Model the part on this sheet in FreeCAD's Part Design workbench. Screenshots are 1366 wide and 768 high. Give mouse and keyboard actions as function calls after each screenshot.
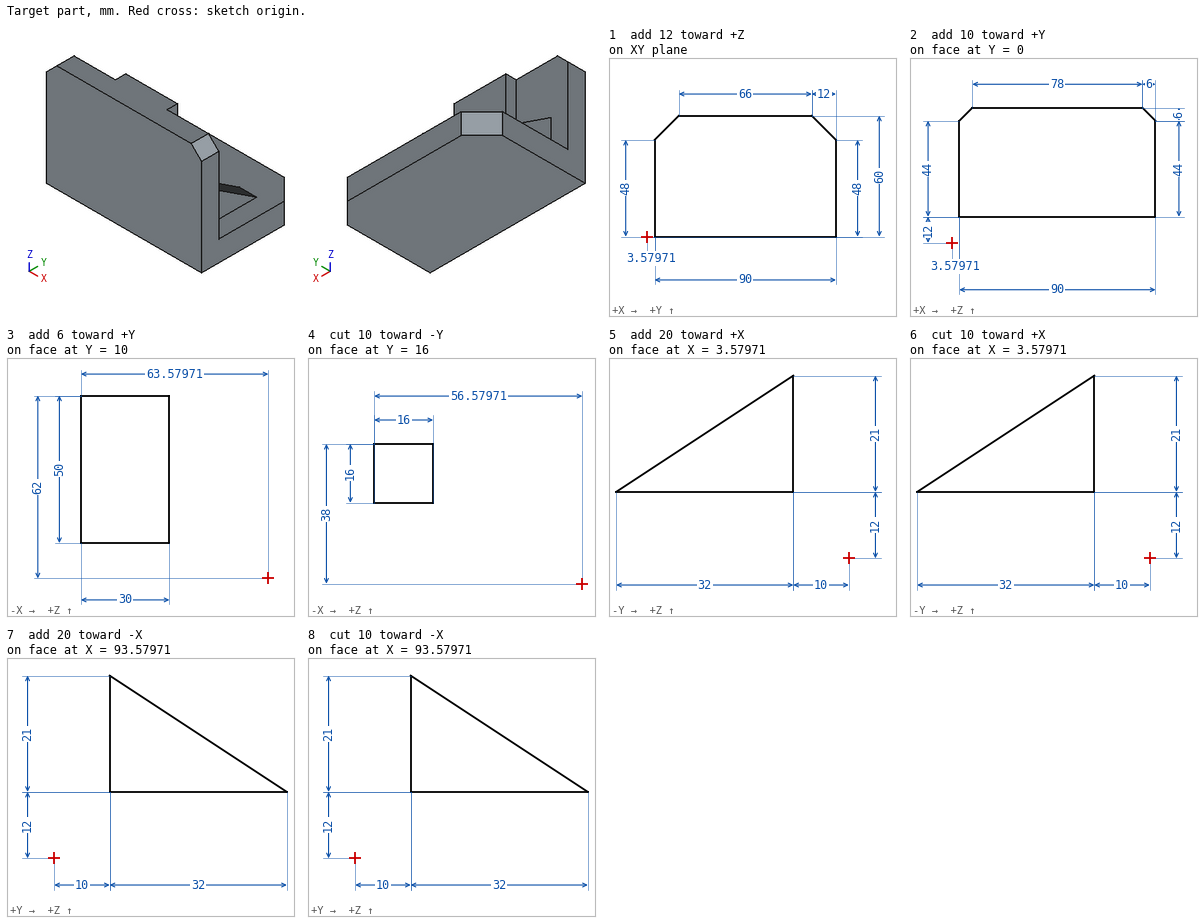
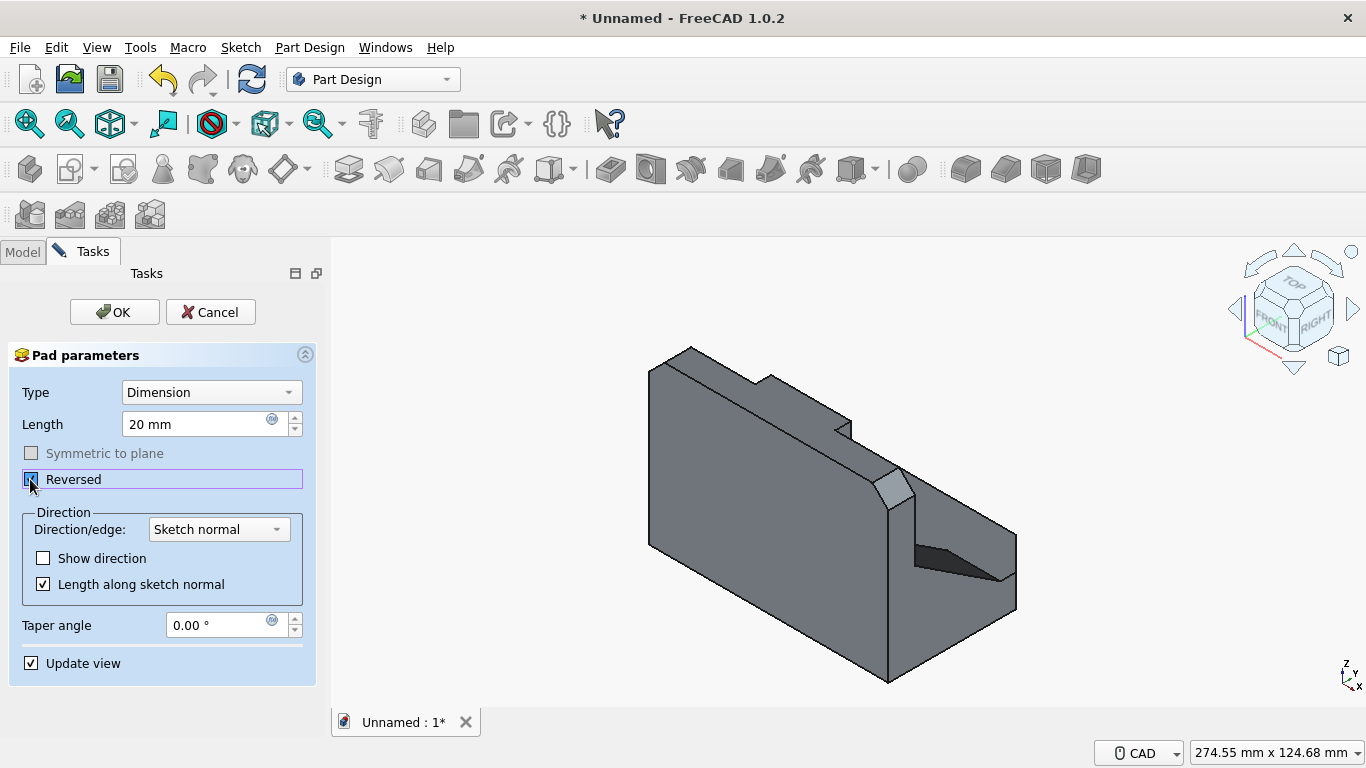
click(115, 312)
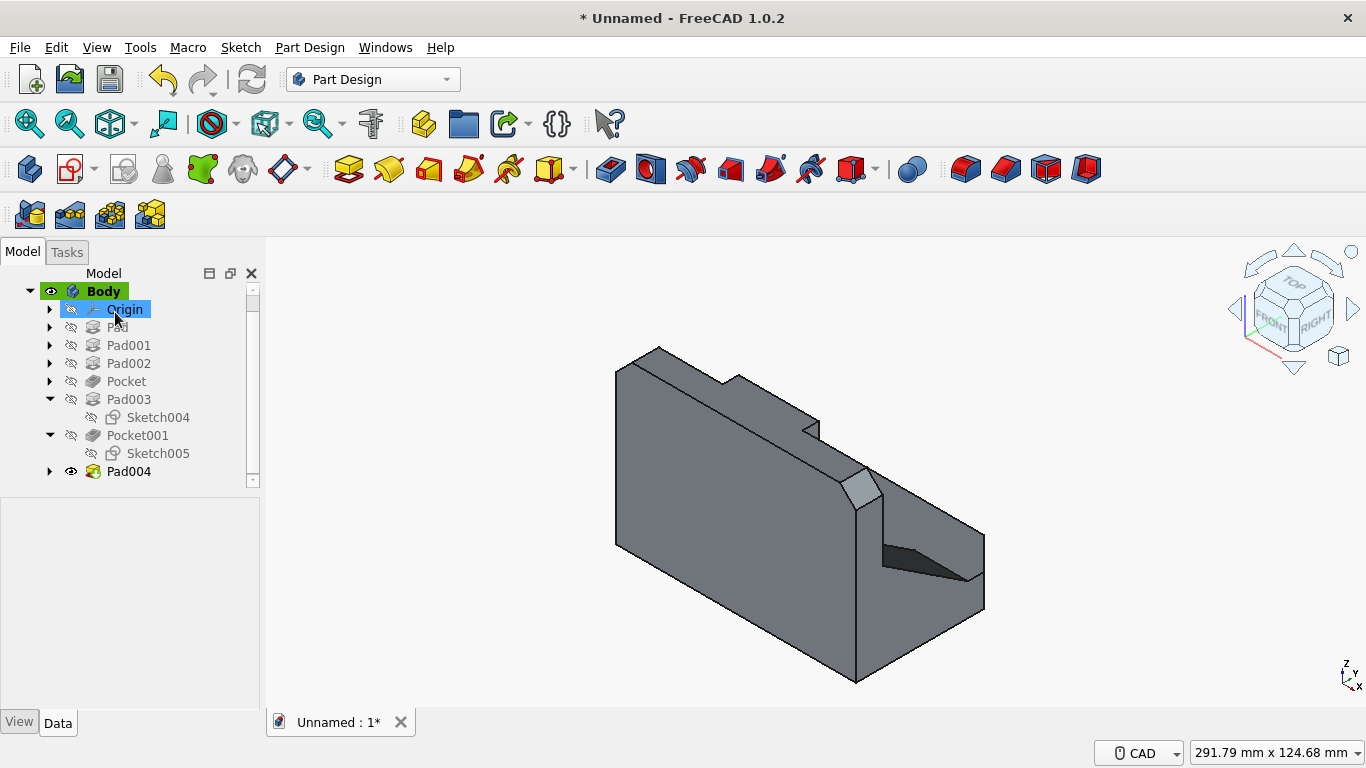
click(902, 619)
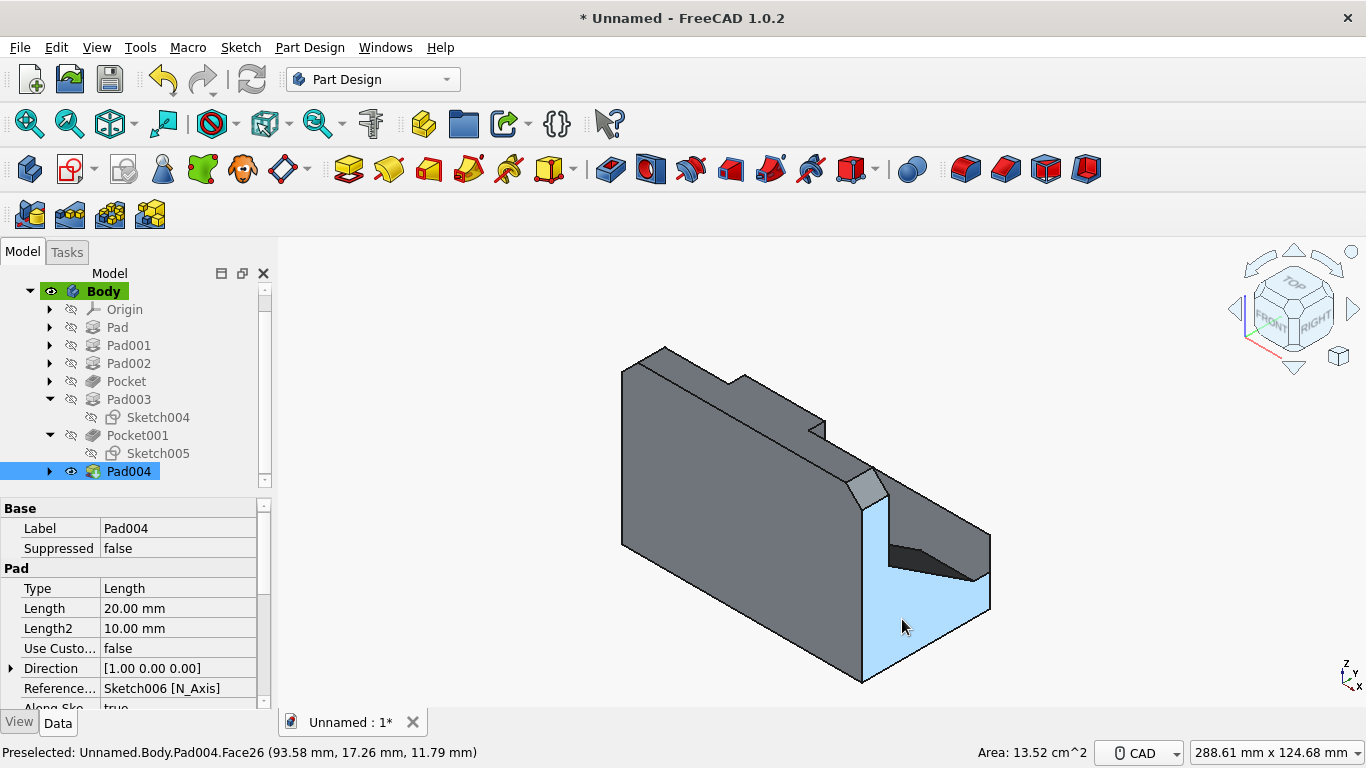
click(70, 170)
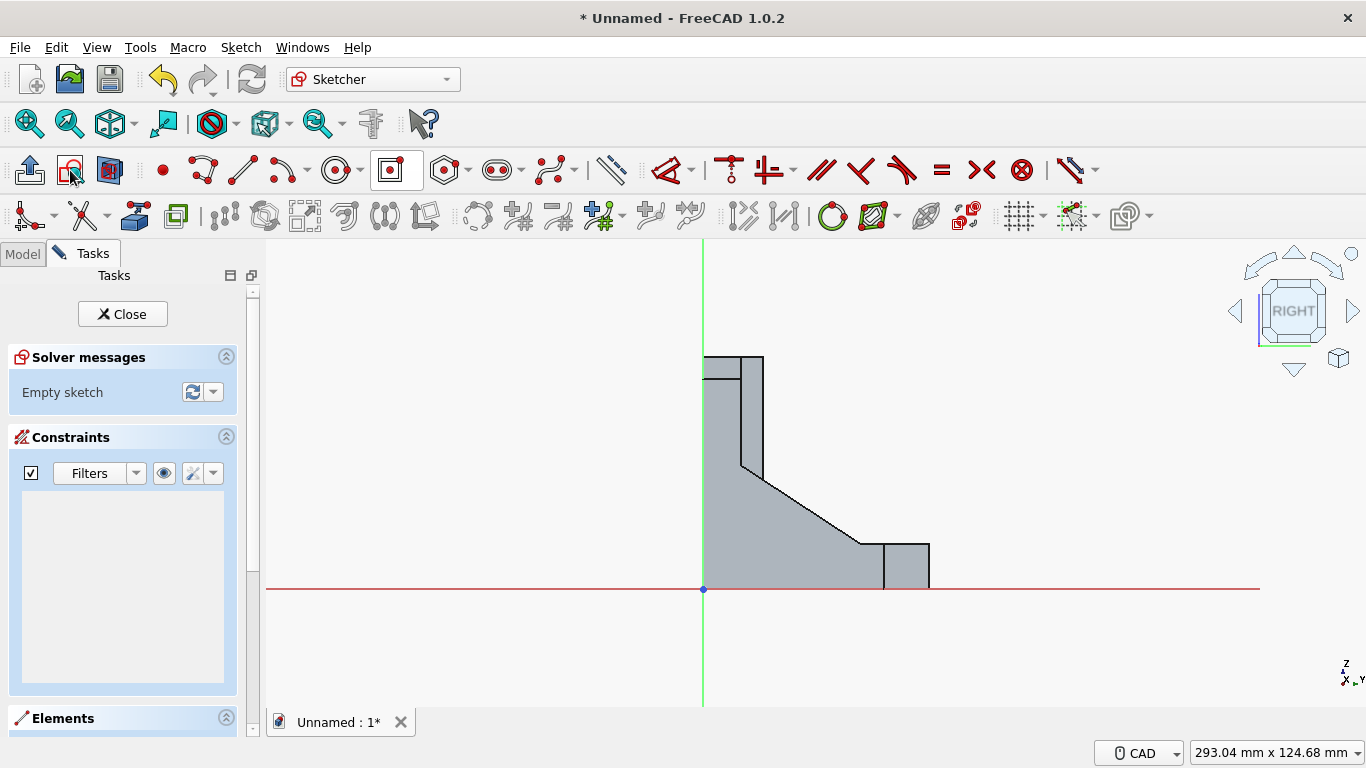
scroll(811, 572, up, 4)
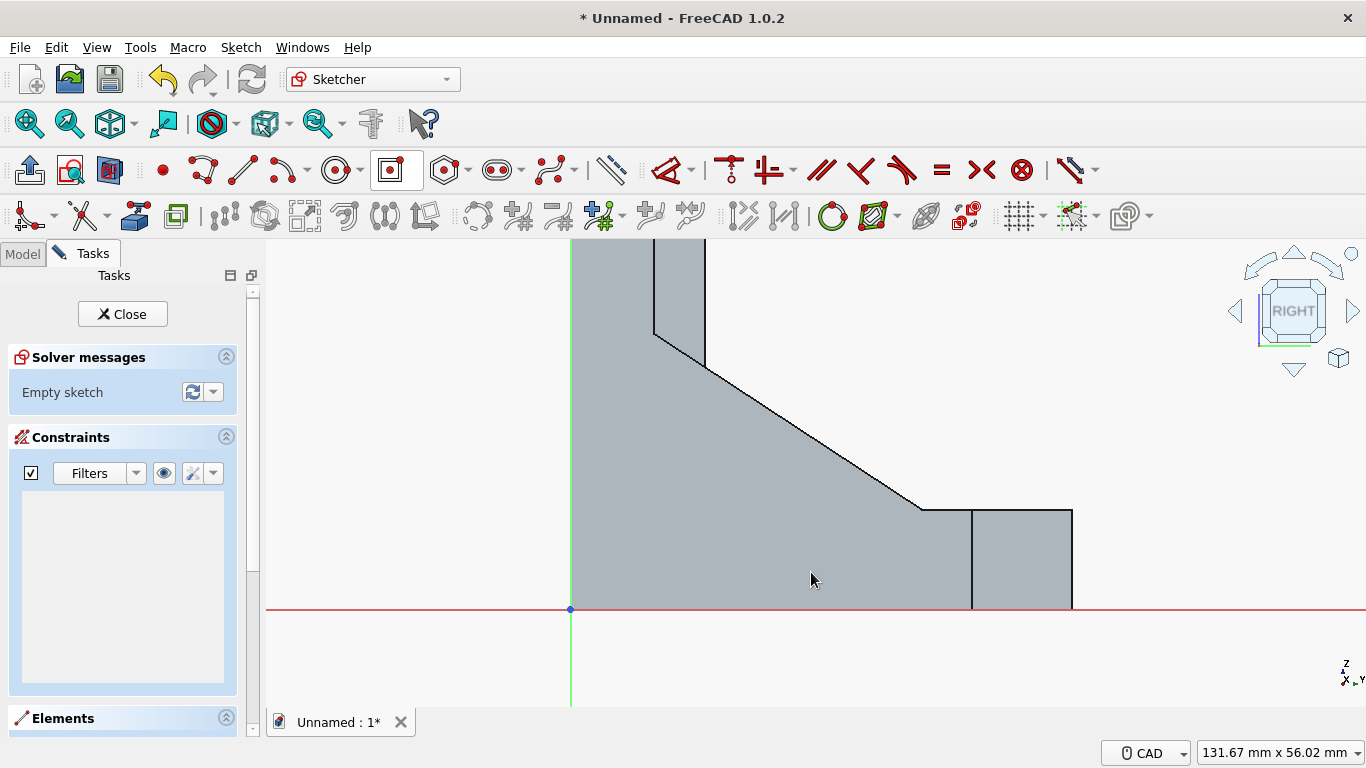
click(204, 170)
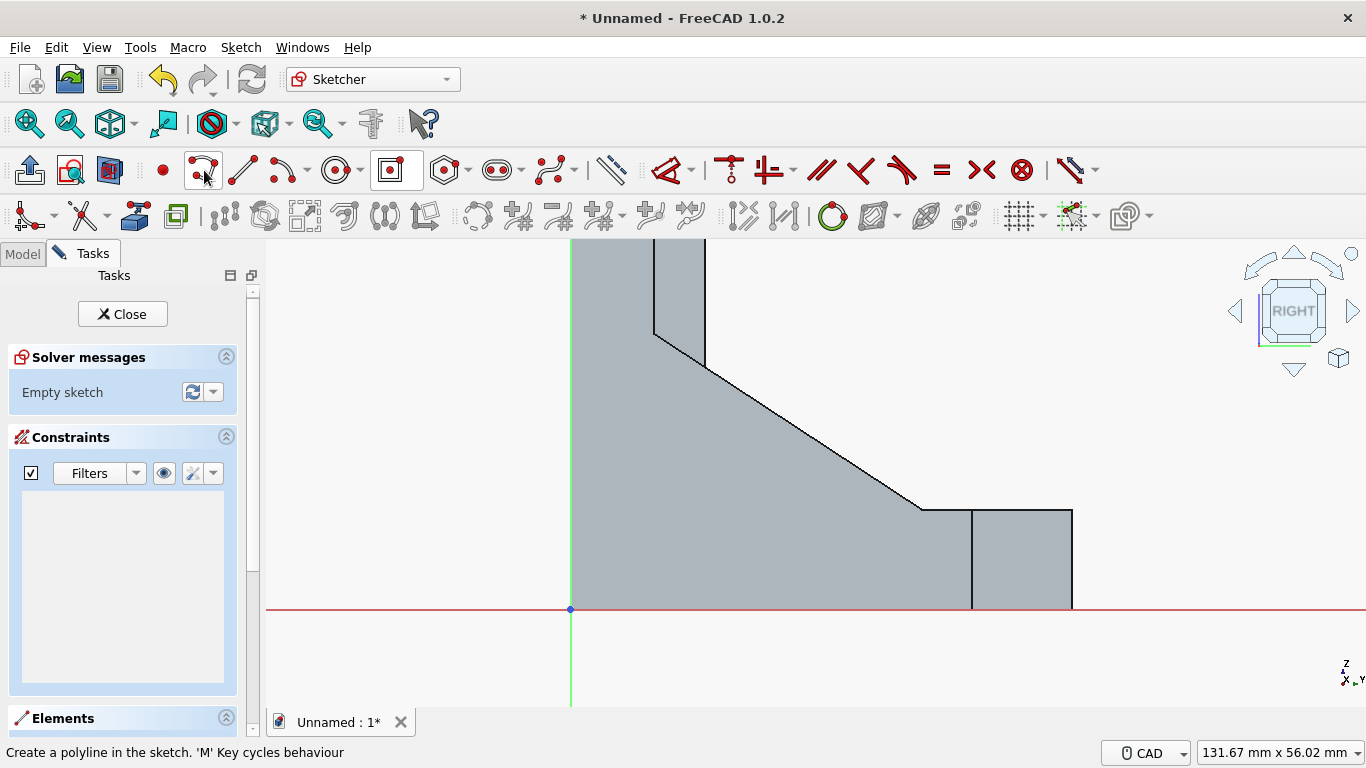
click(654, 510)
click(922, 510)
click(654, 334)
click(654, 511)
key(Escape)
key(Escape)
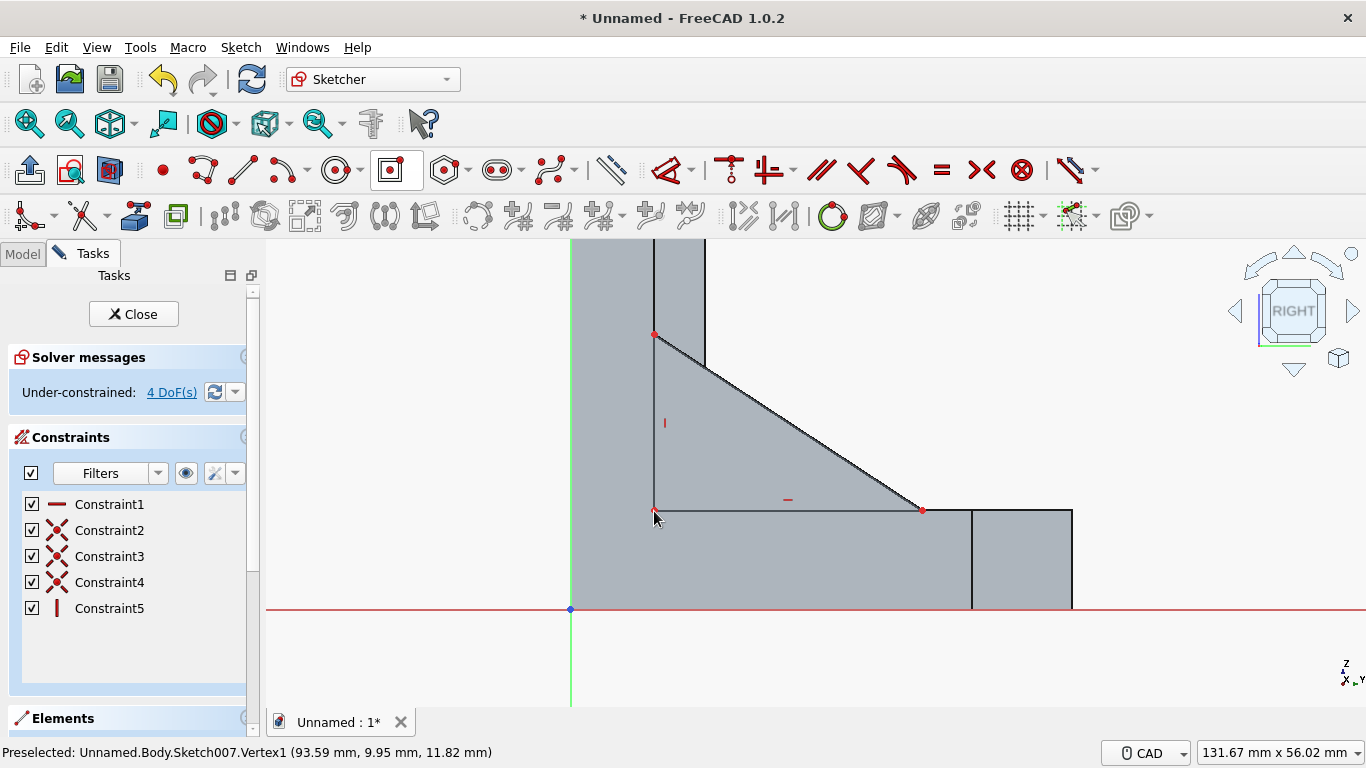
click(666, 170)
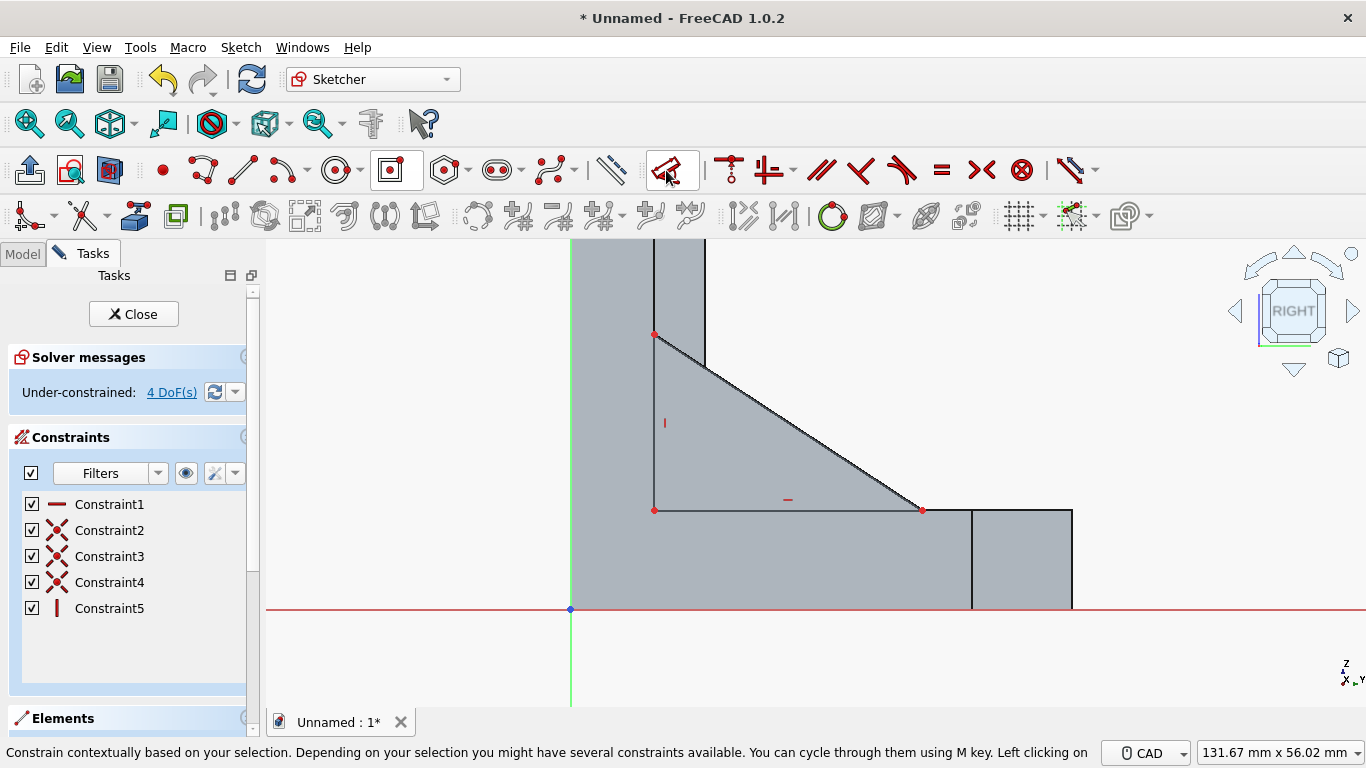
click(734, 511)
click(788, 545)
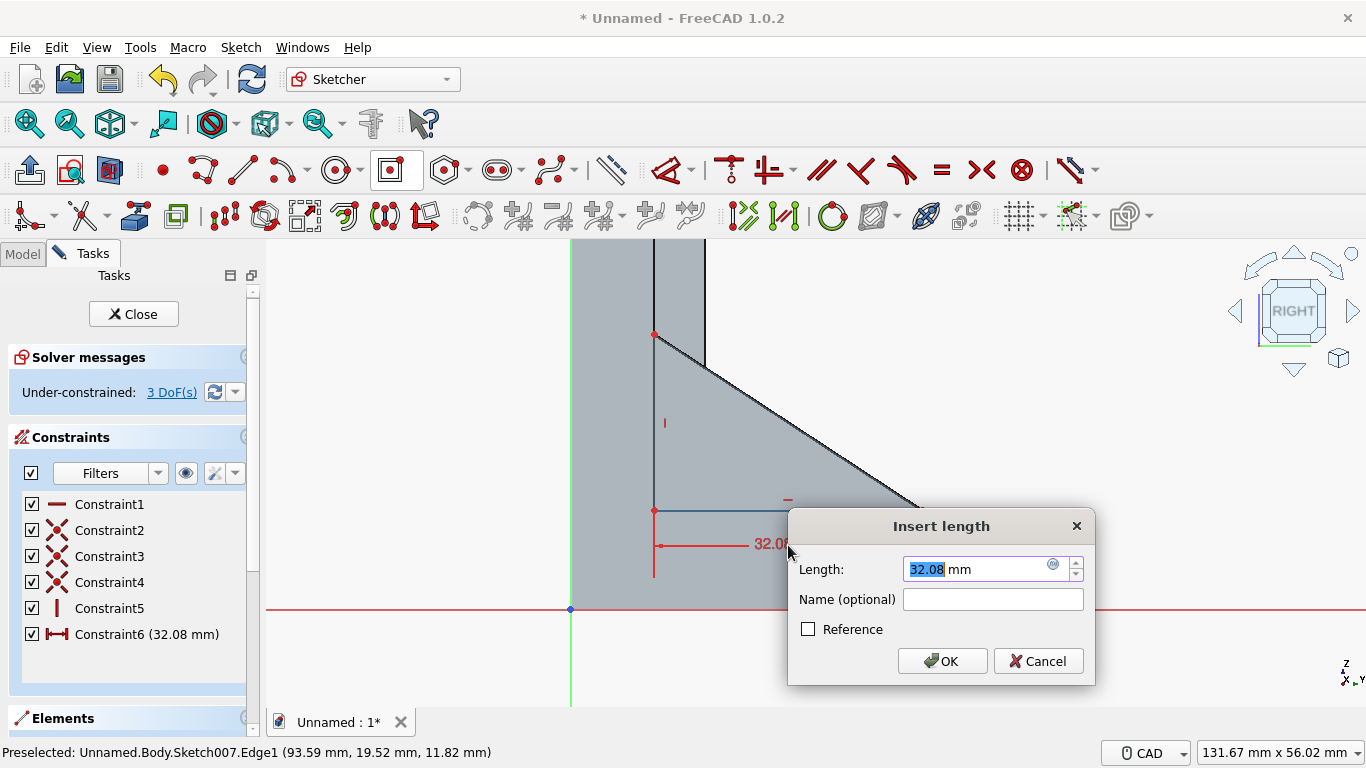
text(32)
key(Return)